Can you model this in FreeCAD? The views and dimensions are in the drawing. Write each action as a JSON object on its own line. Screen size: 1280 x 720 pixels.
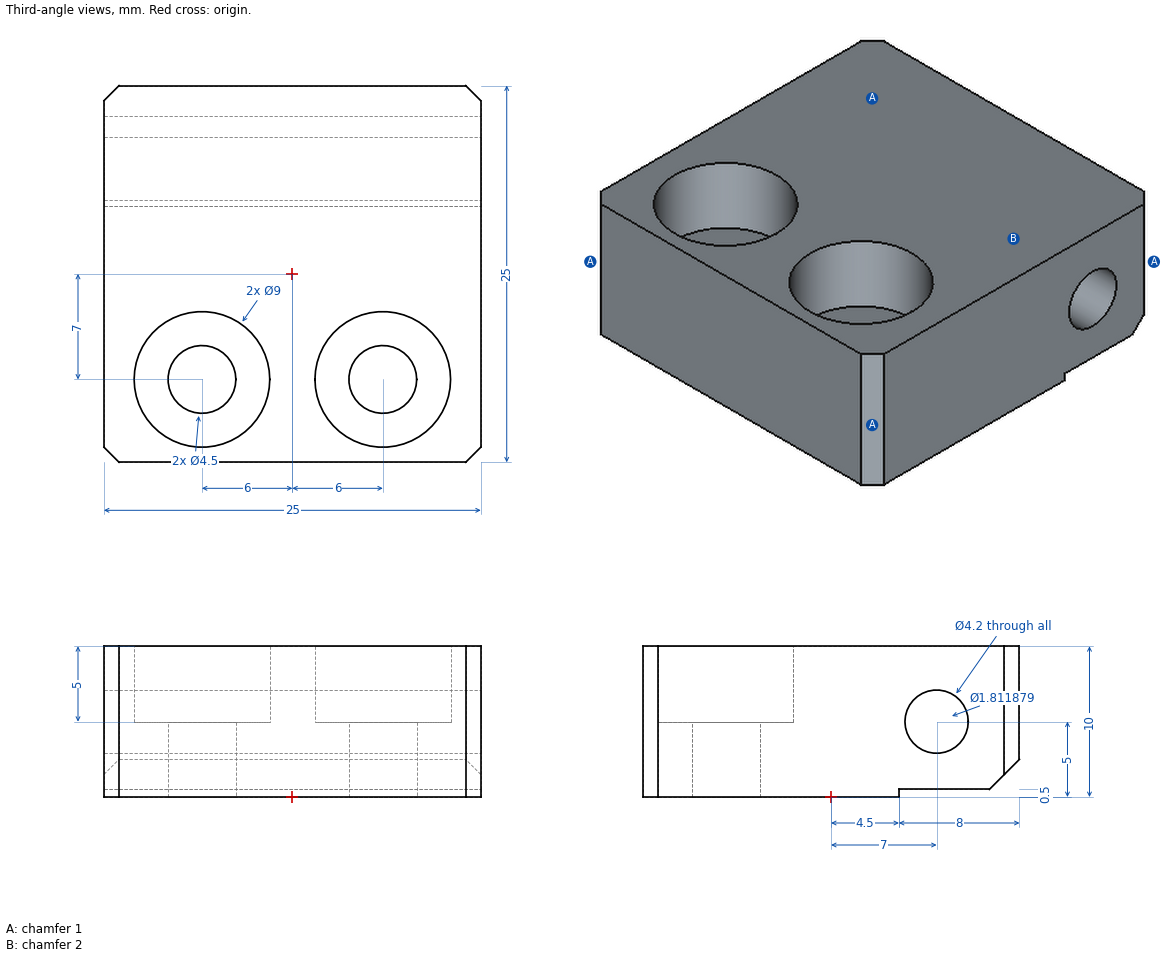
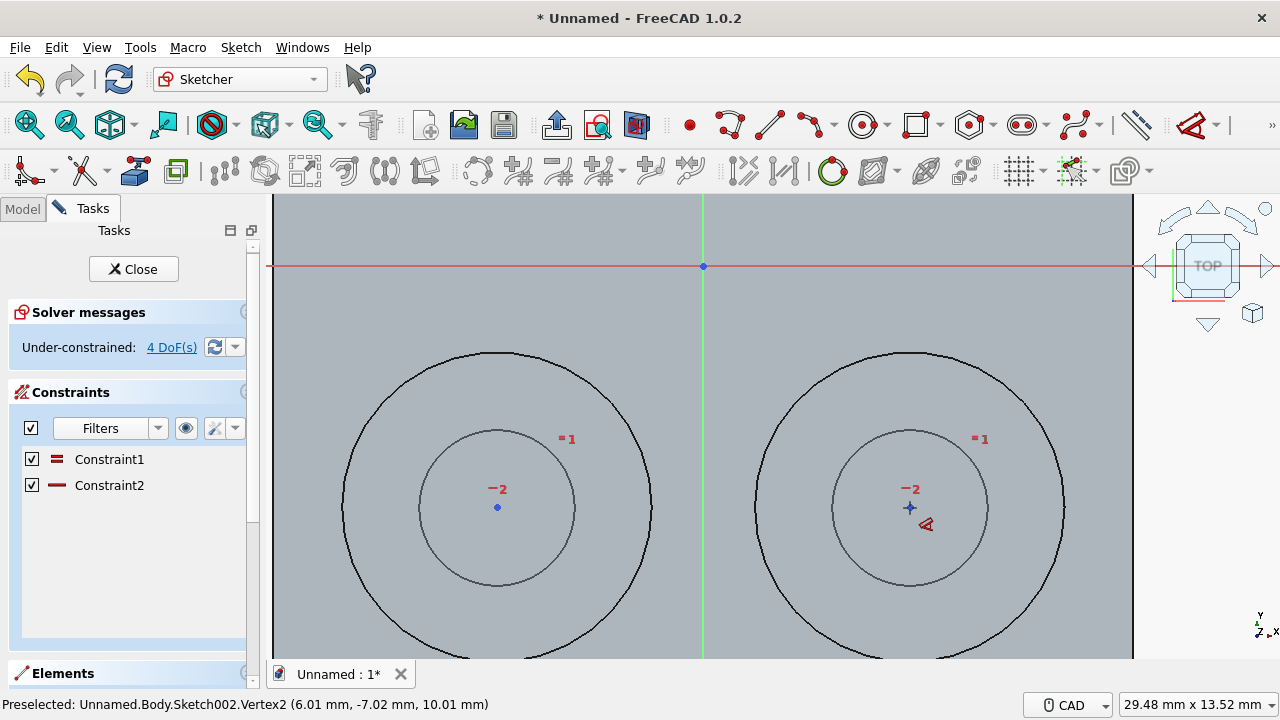
{"action": "left_click", "coordinate": [552, 453]}
{"action": "left_click", "coordinate": [575, 430]}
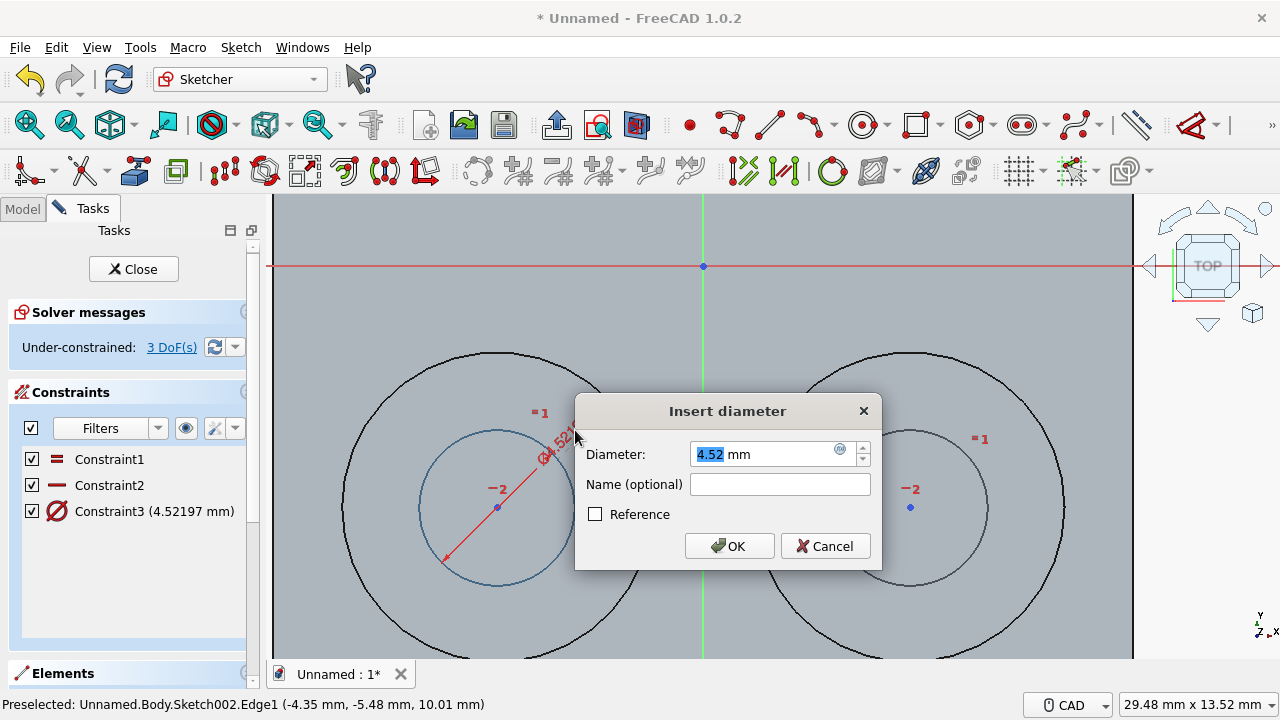
{"action": "type", "text": "4.5"}
{"action": "key", "text": "Return"}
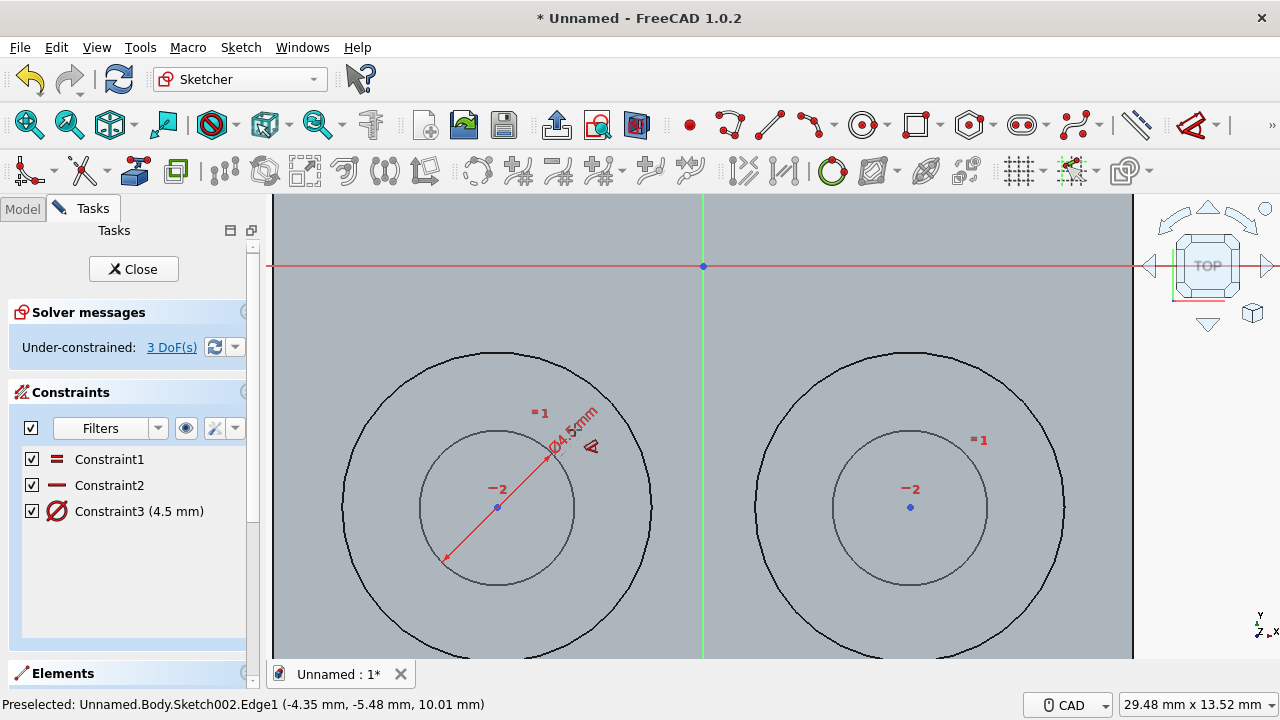
{"action": "left_click", "coordinate": [497, 508]}
{"action": "left_click", "coordinate": [600, 232]}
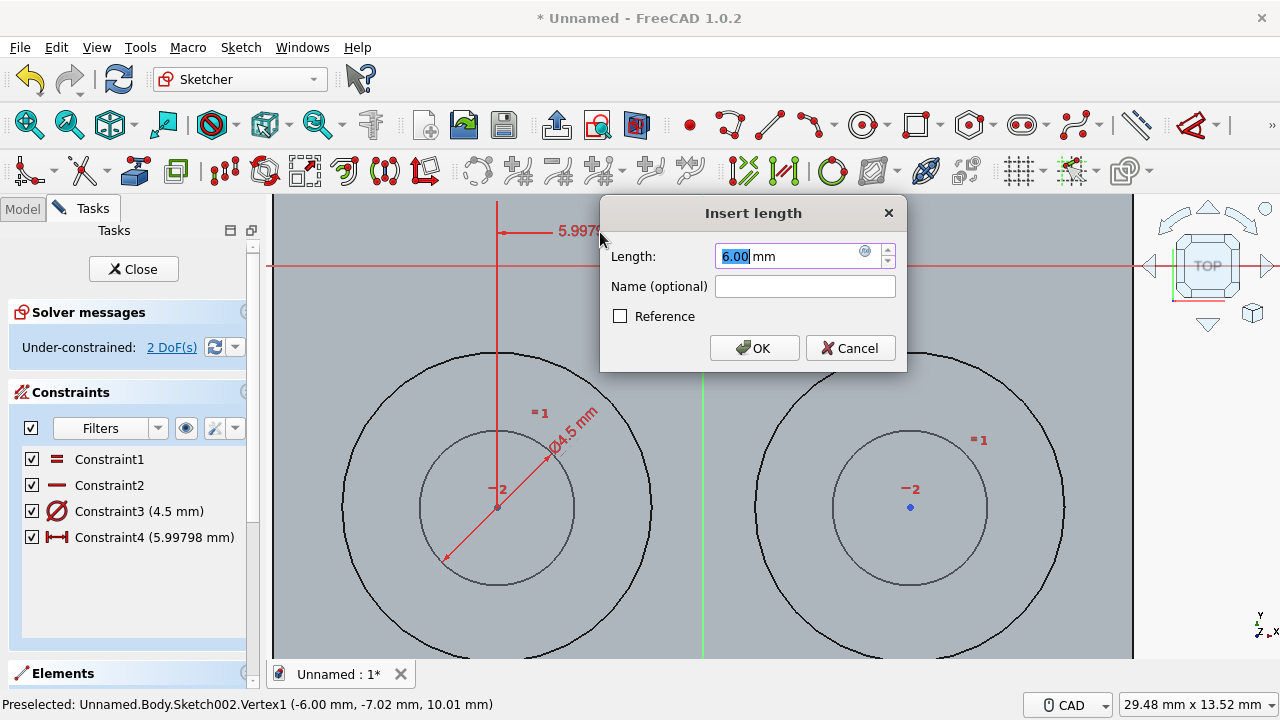
{"action": "type", "text": "6"}
{"action": "key", "text": "Return"}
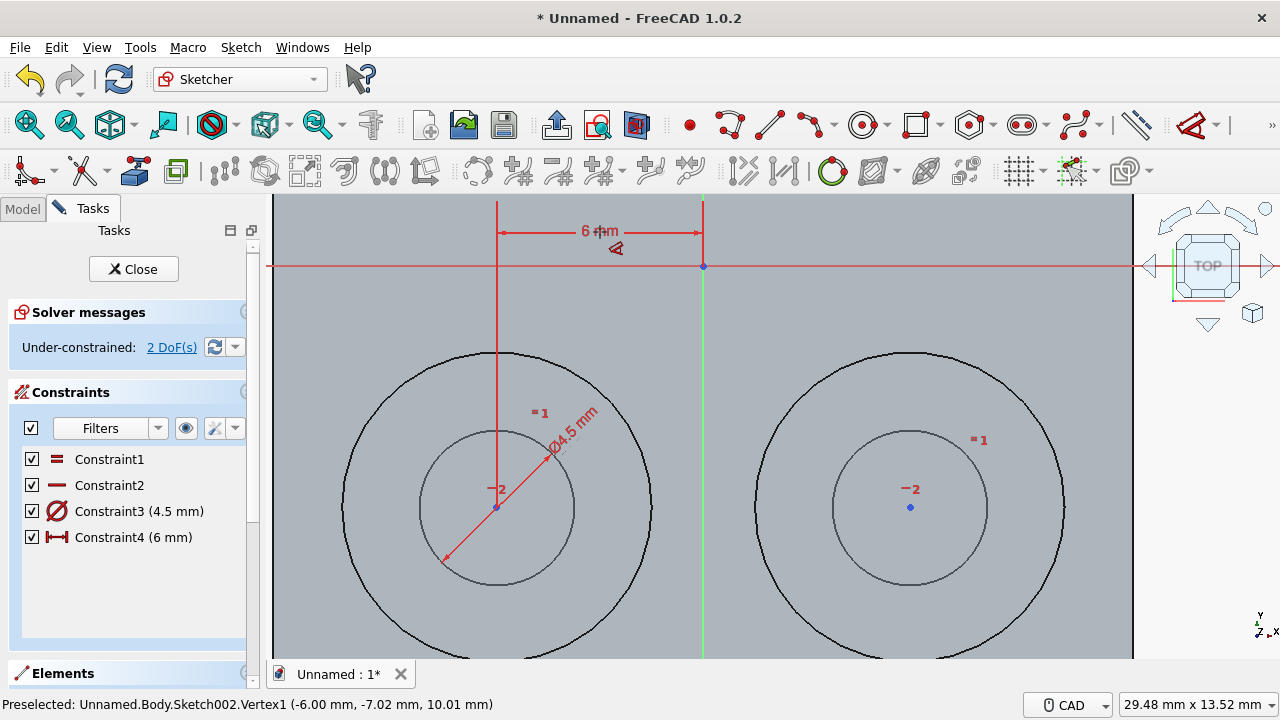
{"action": "left_click", "coordinate": [497, 508]}
{"action": "left_click", "coordinate": [463, 387]}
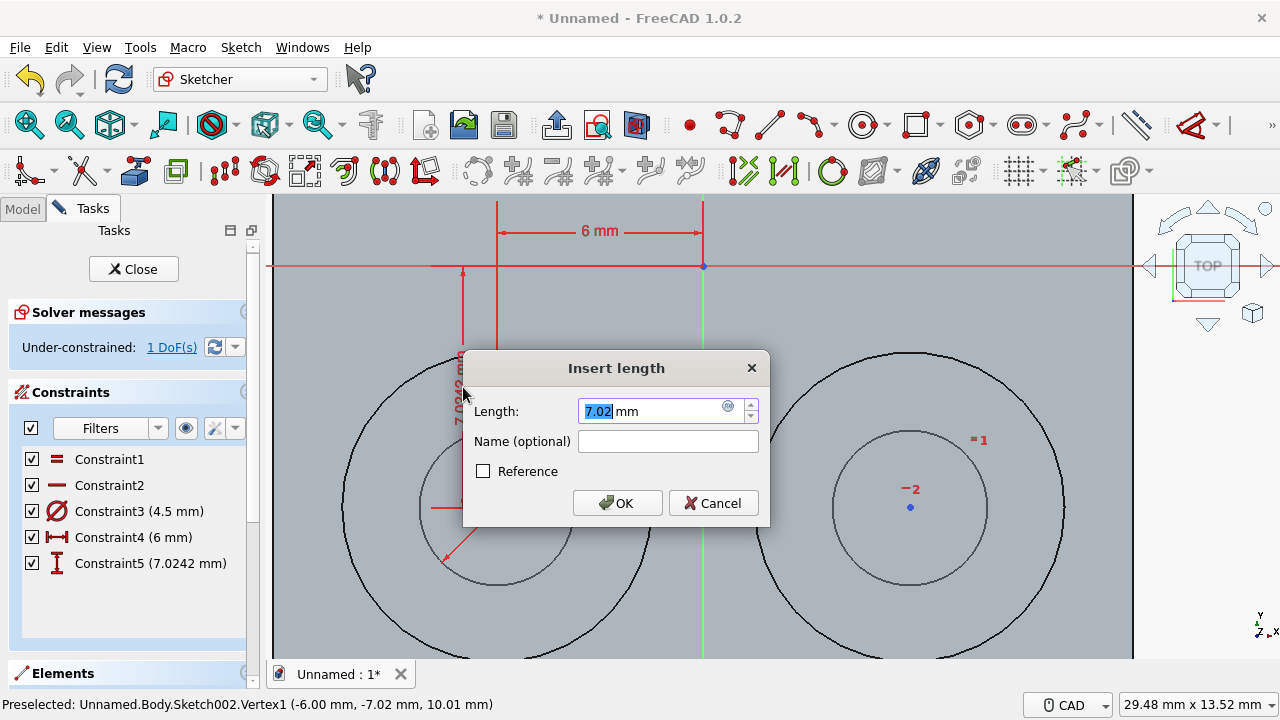
{"action": "type", "text": "7"}
{"action": "key", "text": "Return"}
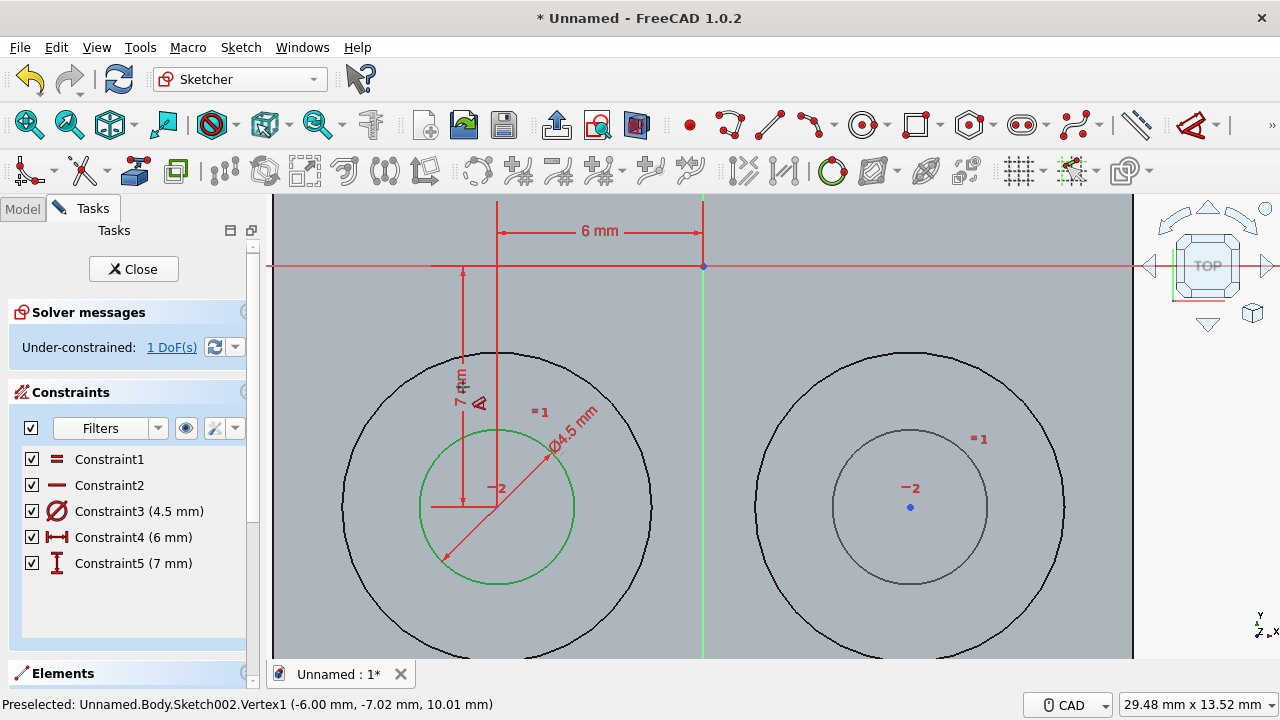
{"action": "left_click", "coordinate": [910, 507]}
{"action": "left_click", "coordinate": [807, 232]}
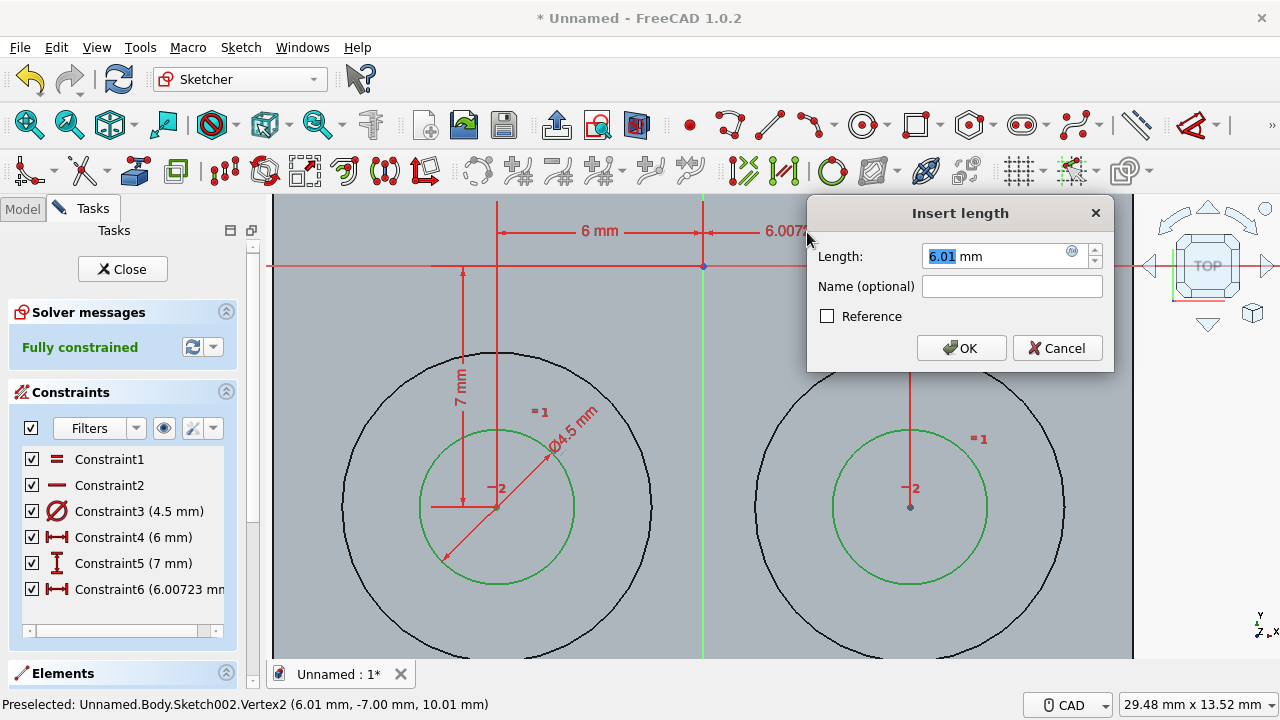
{"action": "type", "text": "6"}
{"action": "key", "text": "Return"}
{"action": "key", "text": "Escape"}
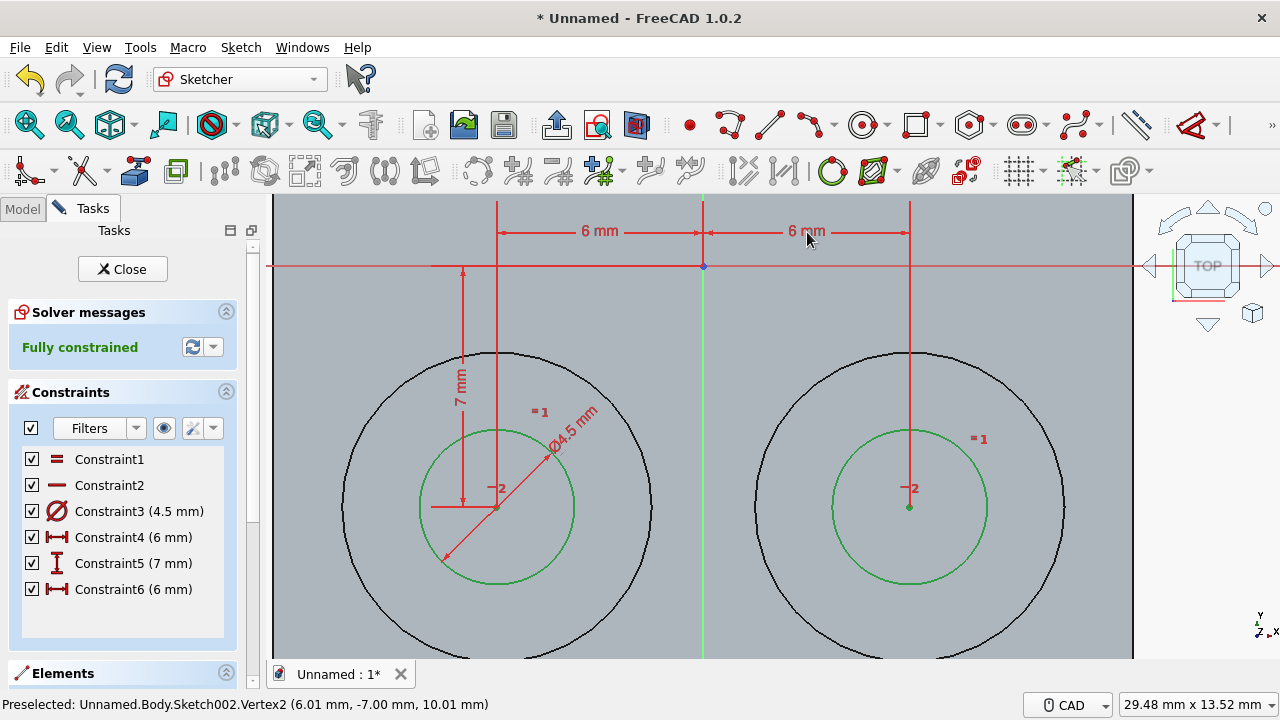
{"action": "left_click", "coordinate": [123, 269]}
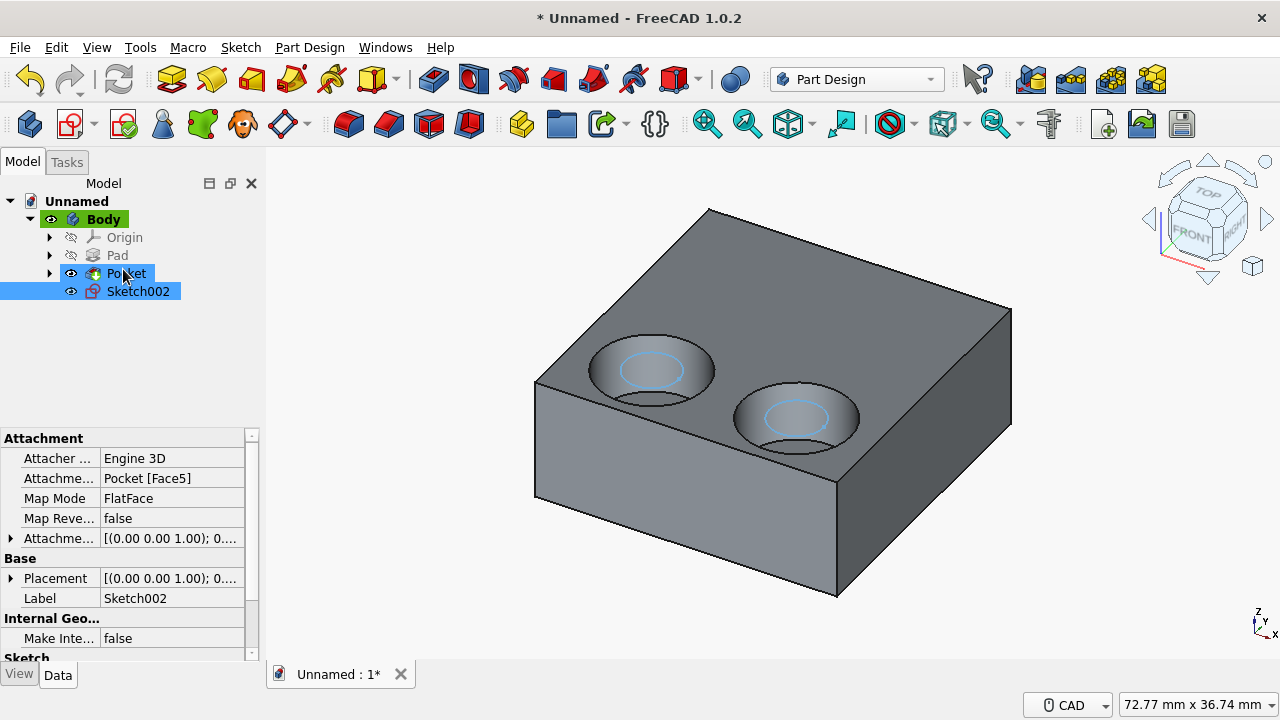
{"action": "left_click", "coordinate": [434, 80]}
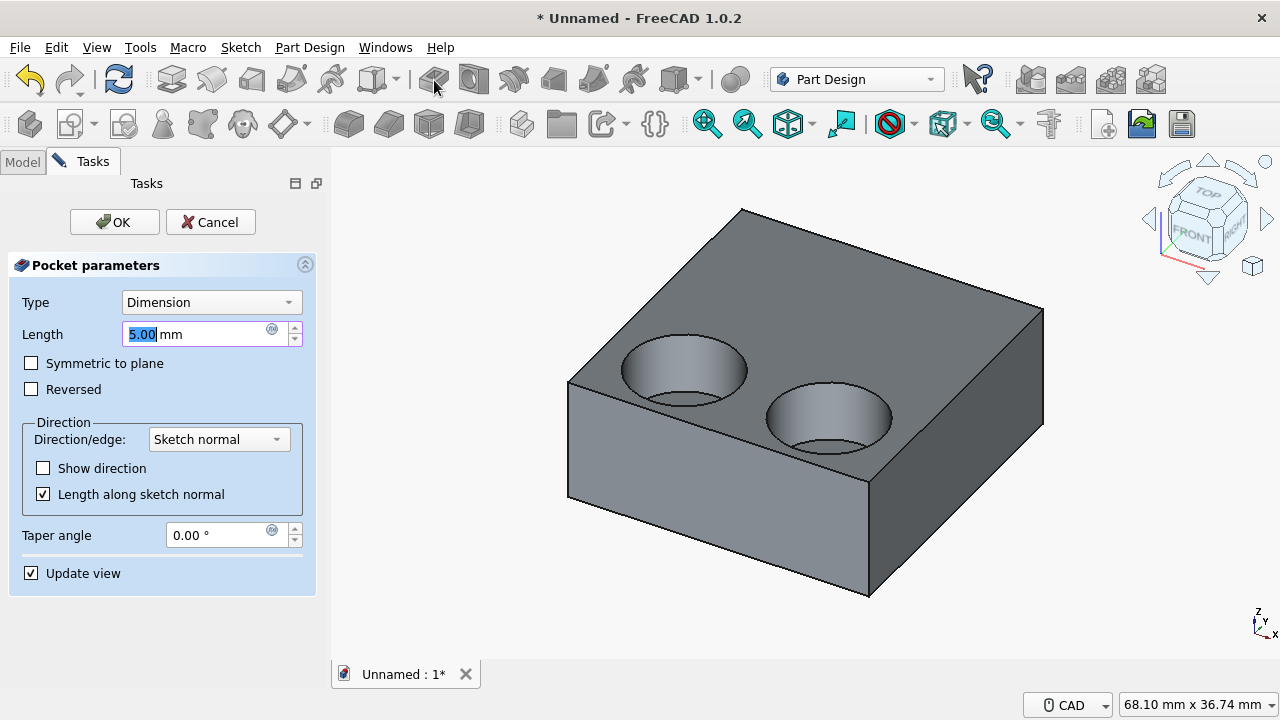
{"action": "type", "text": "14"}
{"action": "key", "text": "Tab"}